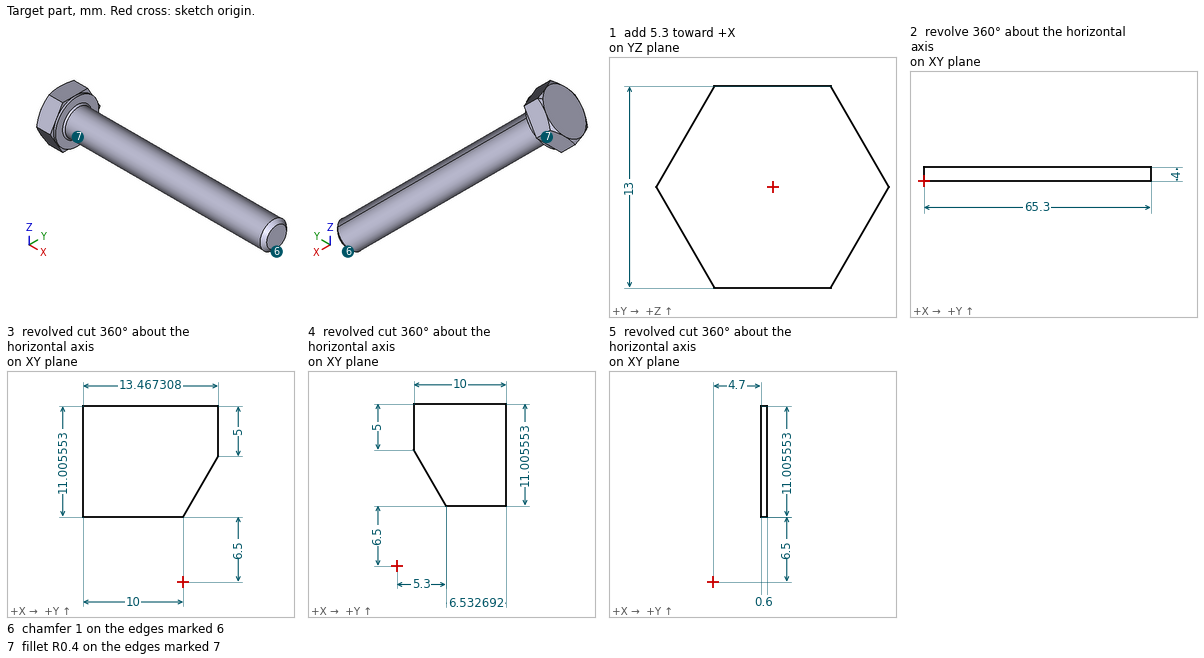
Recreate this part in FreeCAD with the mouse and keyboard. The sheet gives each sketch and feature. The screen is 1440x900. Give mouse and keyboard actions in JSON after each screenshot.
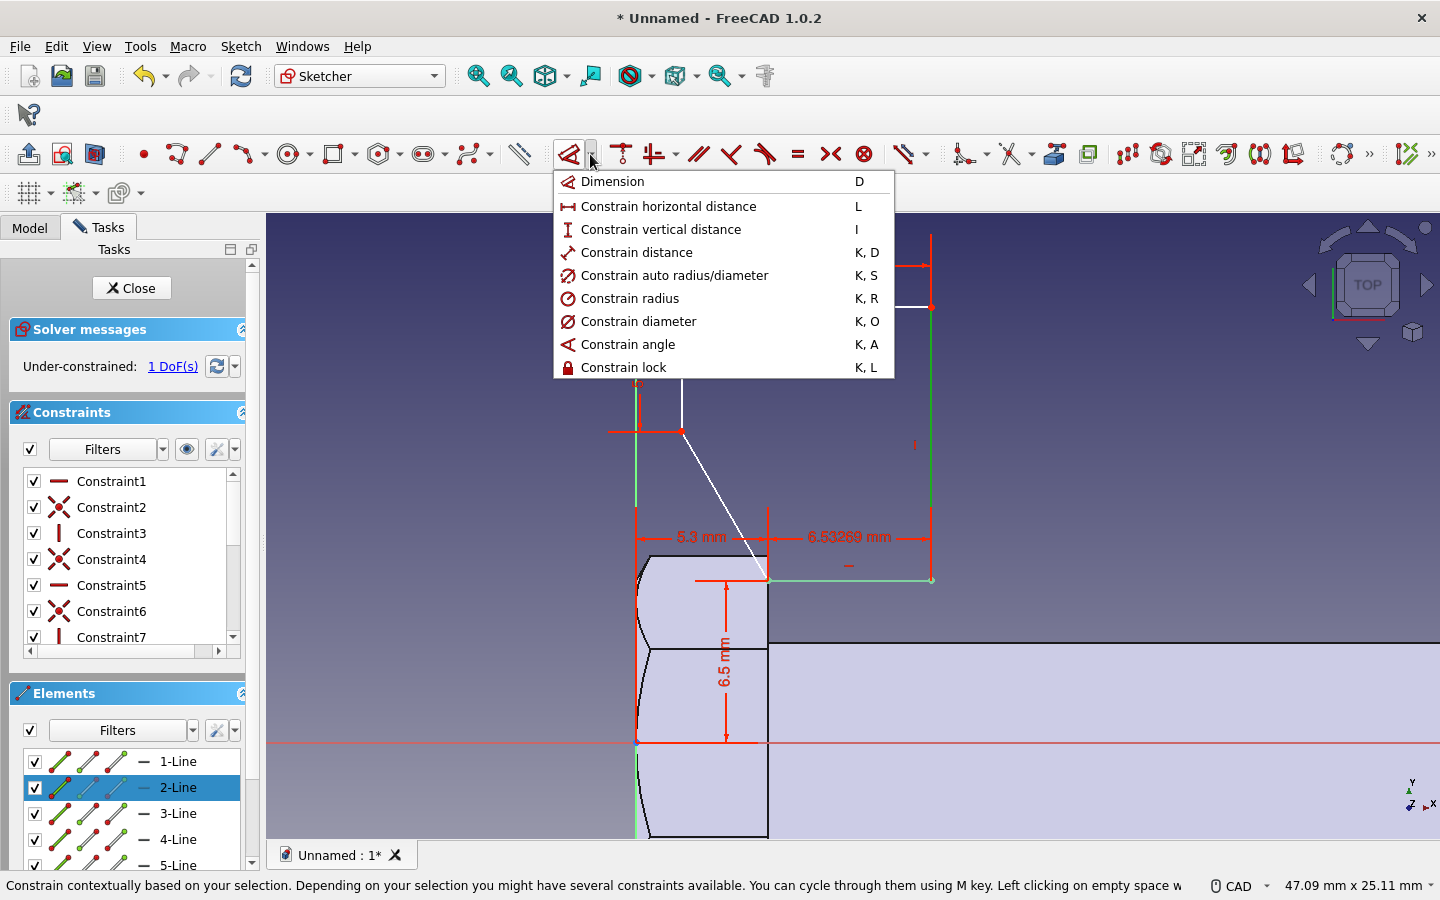
{"action": "left_click", "coordinate": [724, 230]}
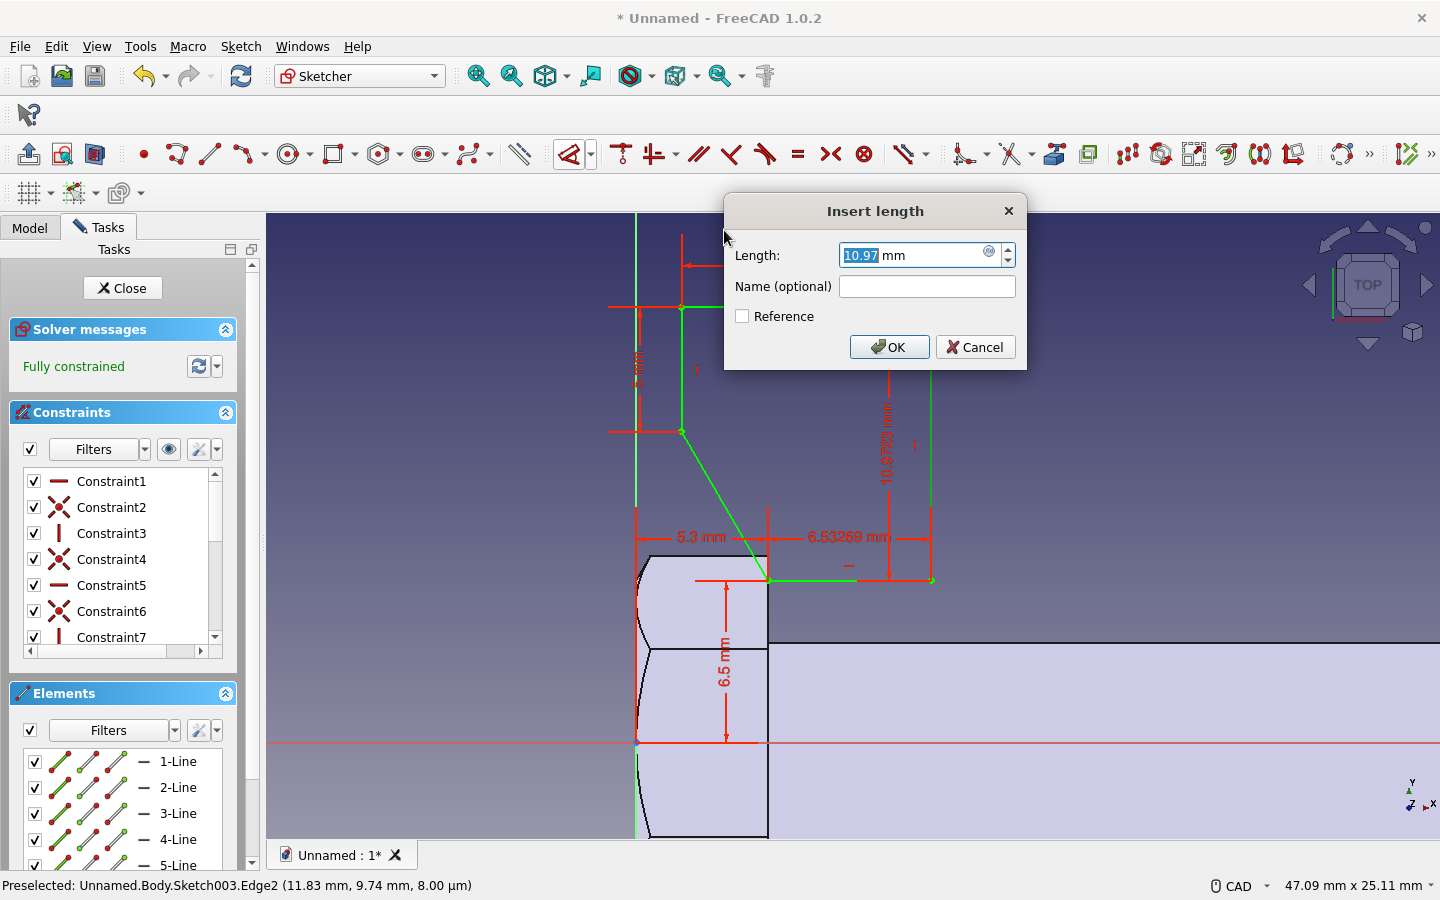
{"action": "type", "text": "11.005553"}
{"action": "key", "text": "Return"}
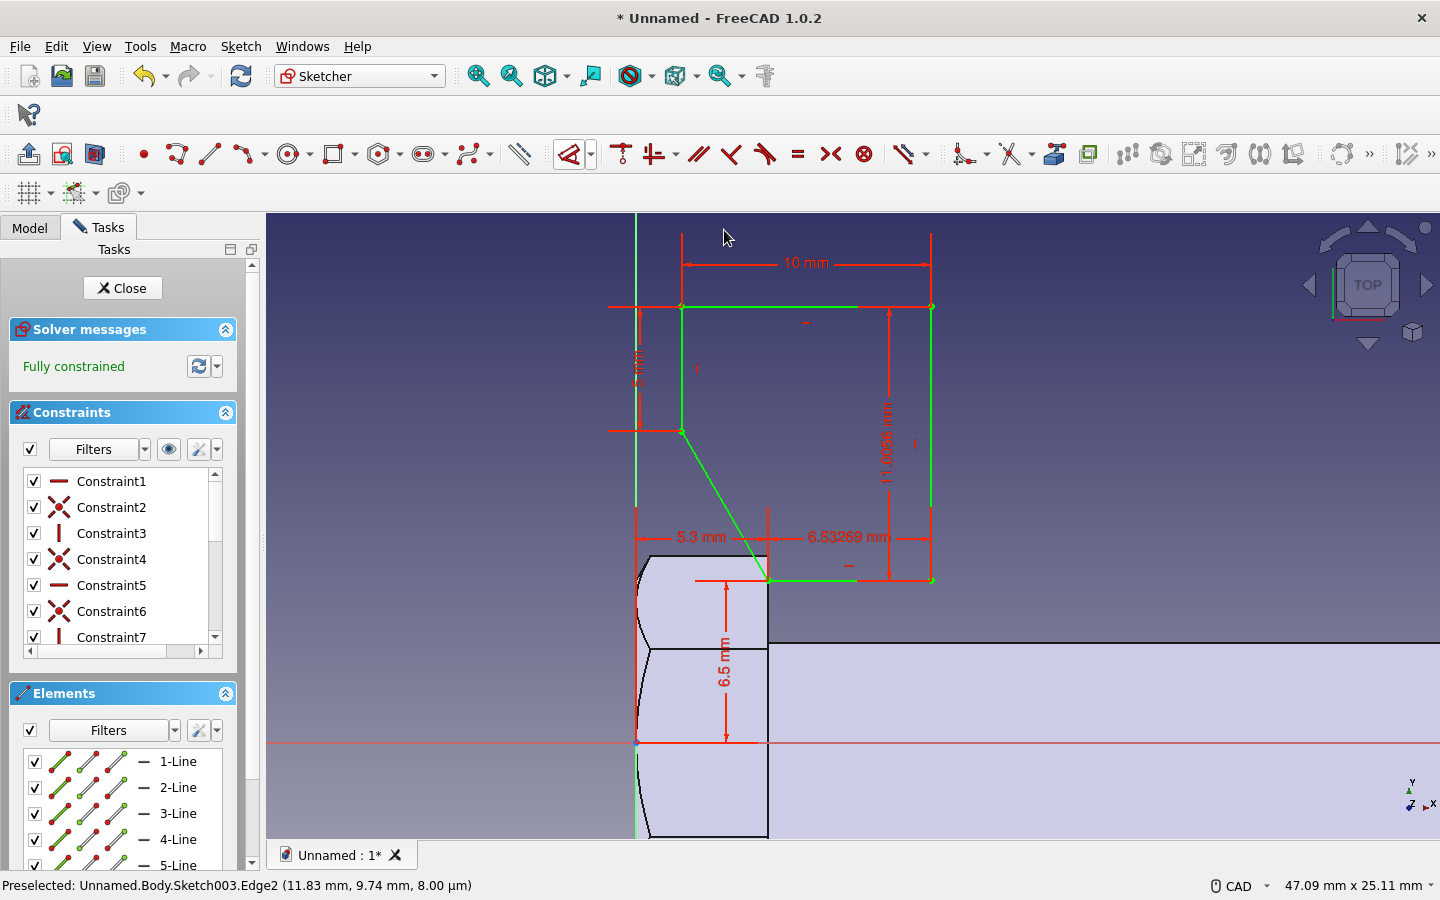
{"action": "left_click", "coordinate": [123, 288]}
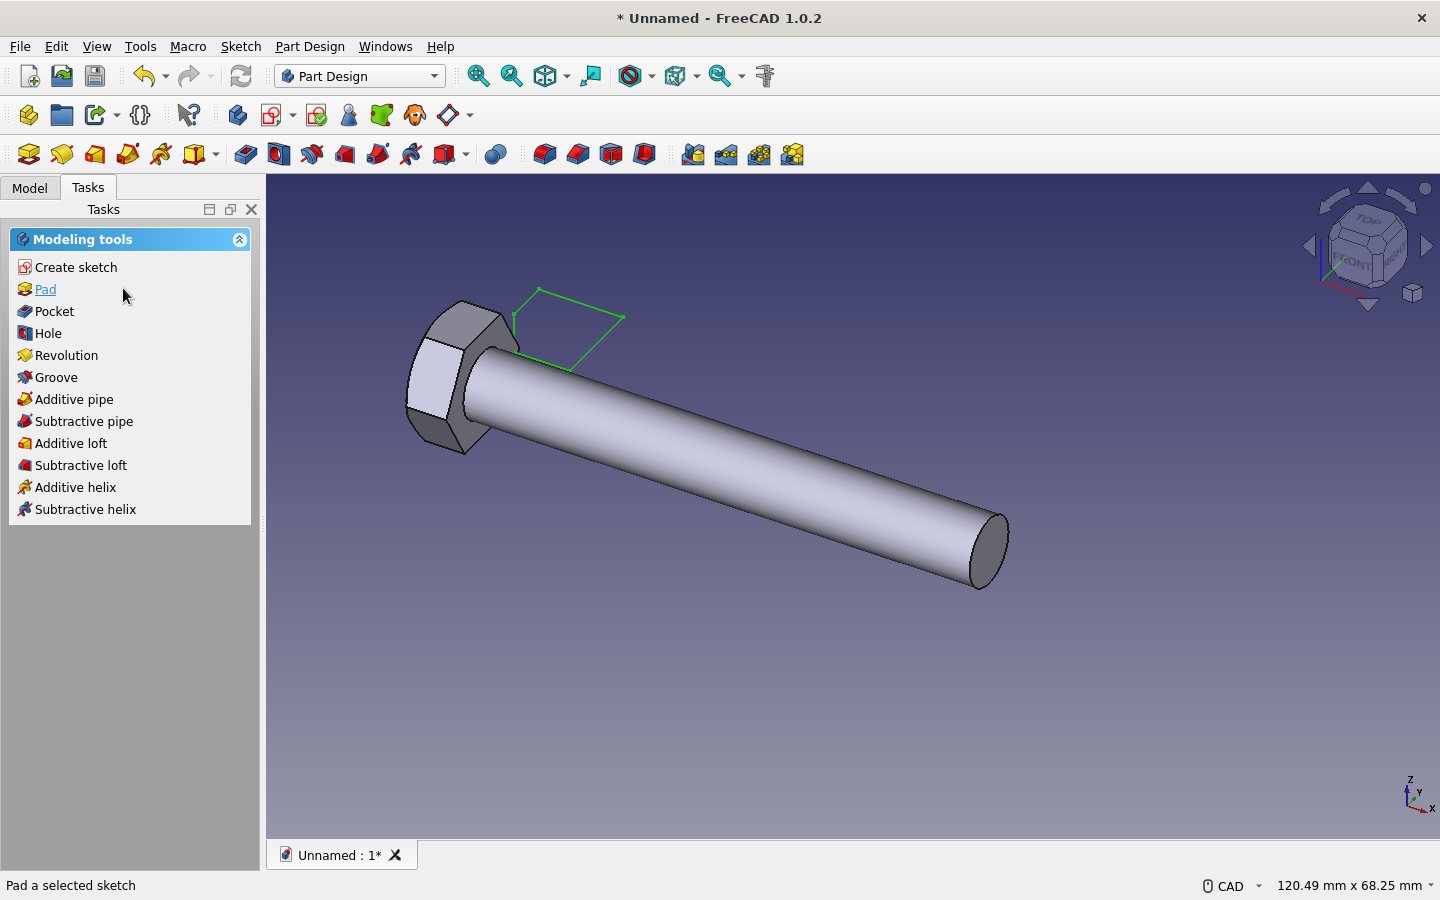
{"action": "left_click", "coordinate": [312, 154]}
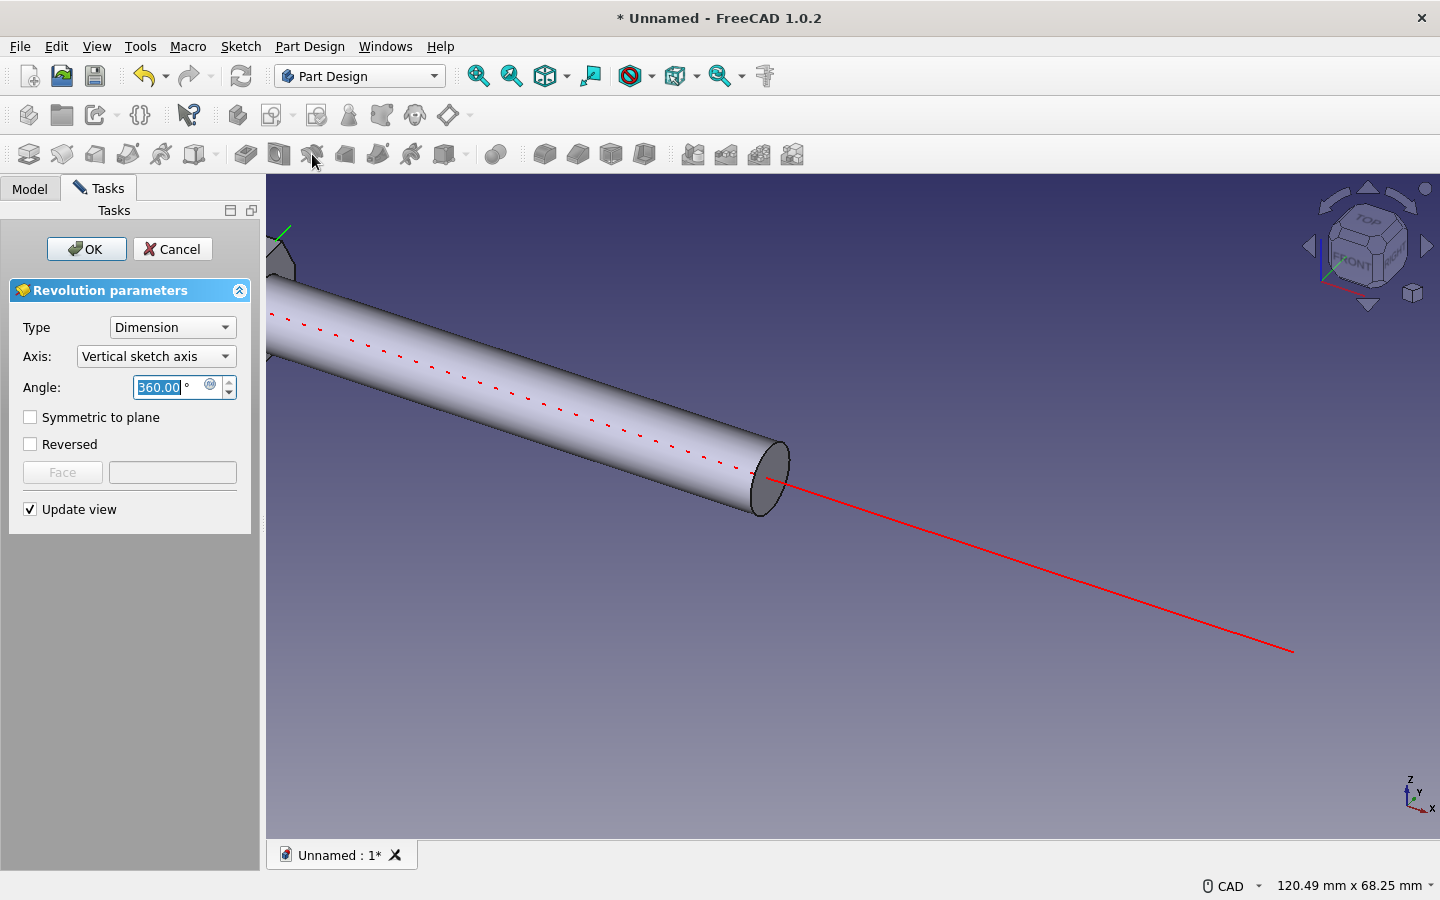
{"action": "left_click", "coordinate": [157, 356]}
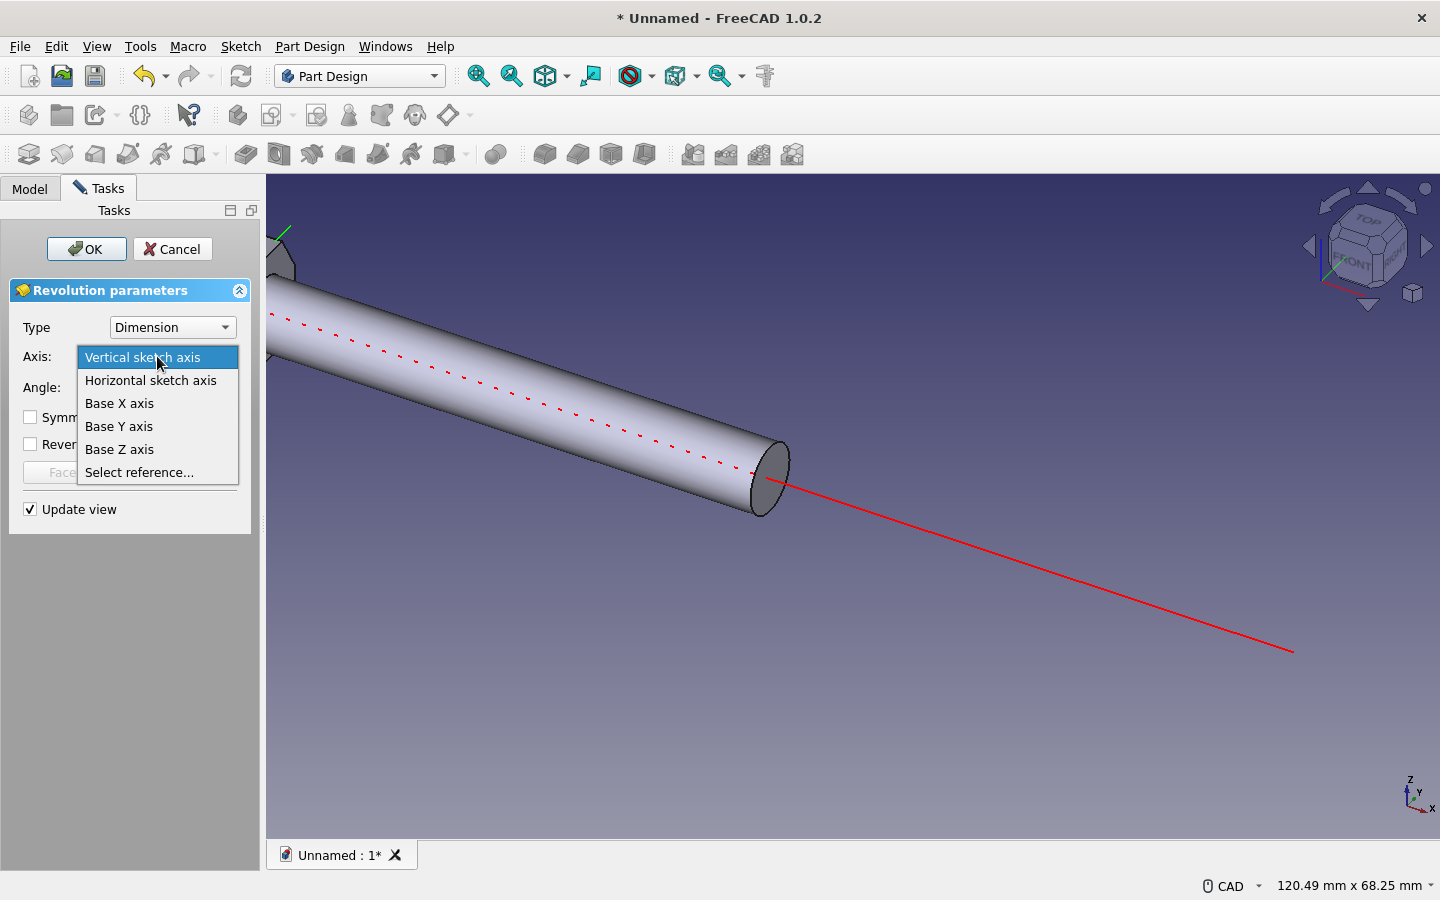
{"action": "left_click", "coordinate": [156, 380]}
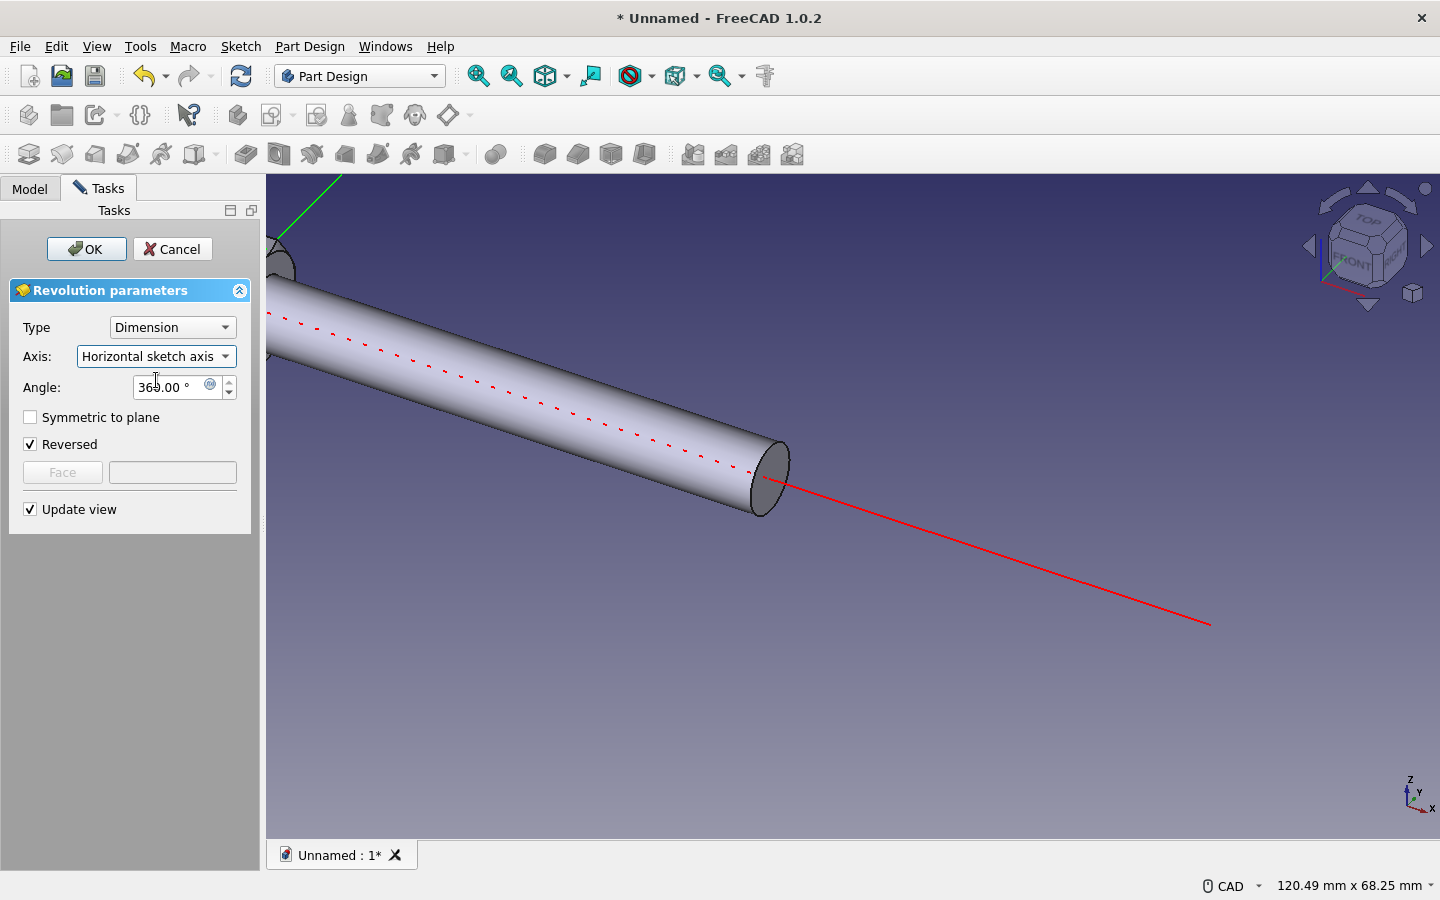
{"action": "left_click", "coordinate": [87, 249]}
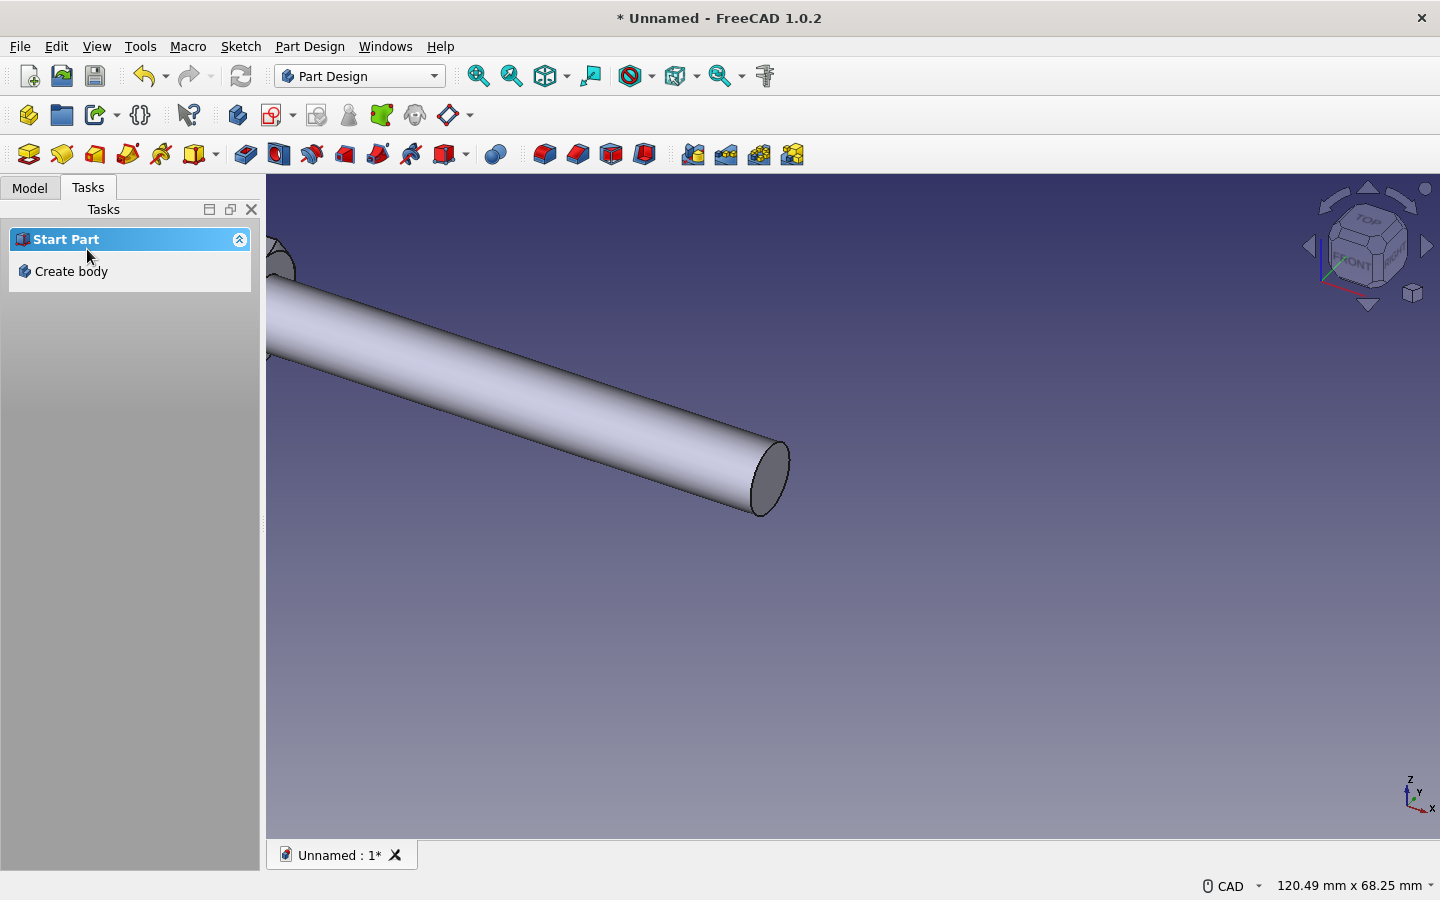
{"action": "left_click", "coordinate": [479, 76]}